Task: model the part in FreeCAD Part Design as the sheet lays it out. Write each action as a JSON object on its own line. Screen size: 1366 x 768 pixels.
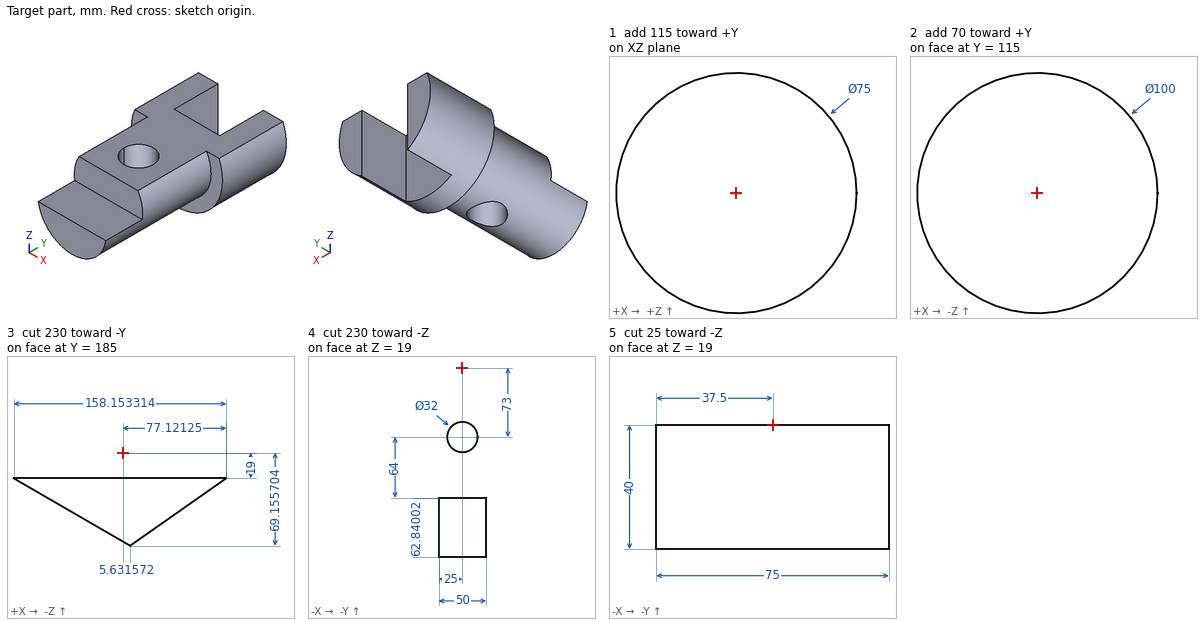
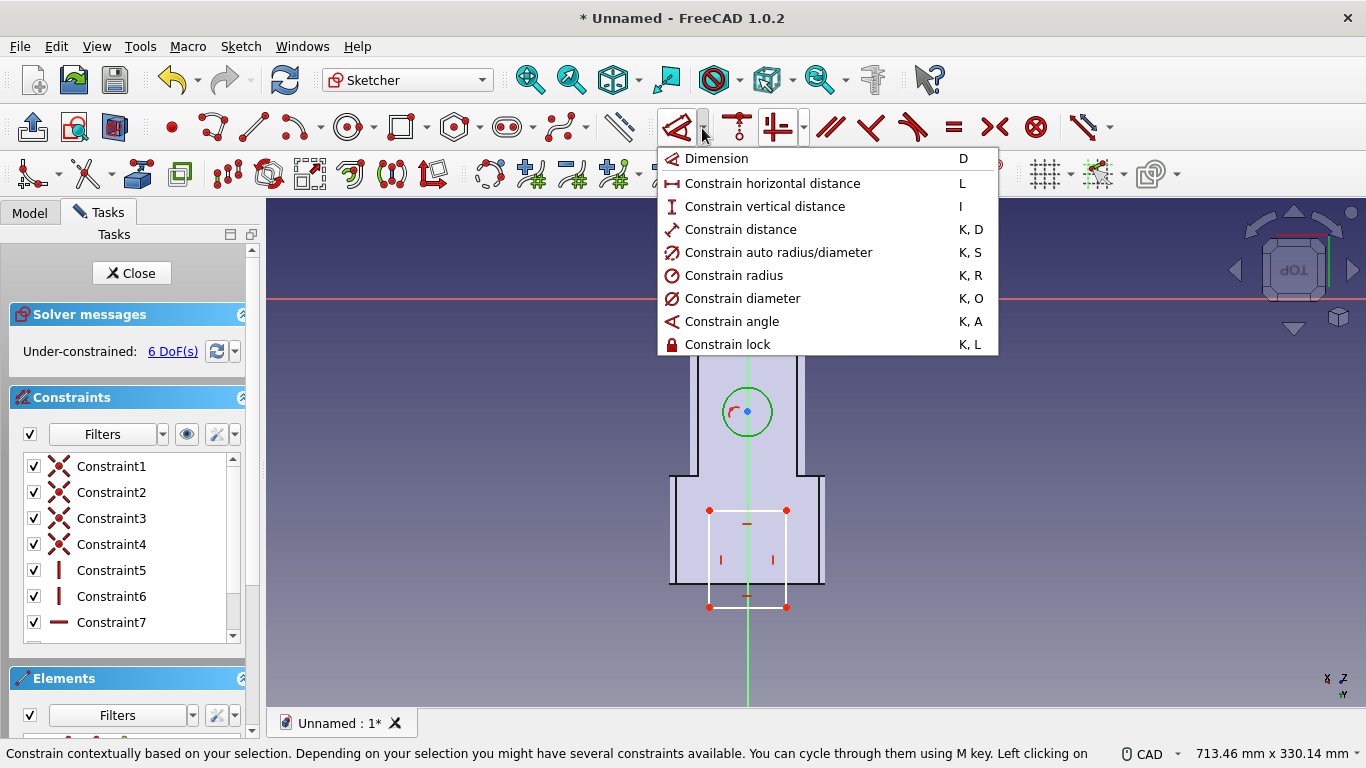
{"action": "left_click", "coordinate": [828, 298]}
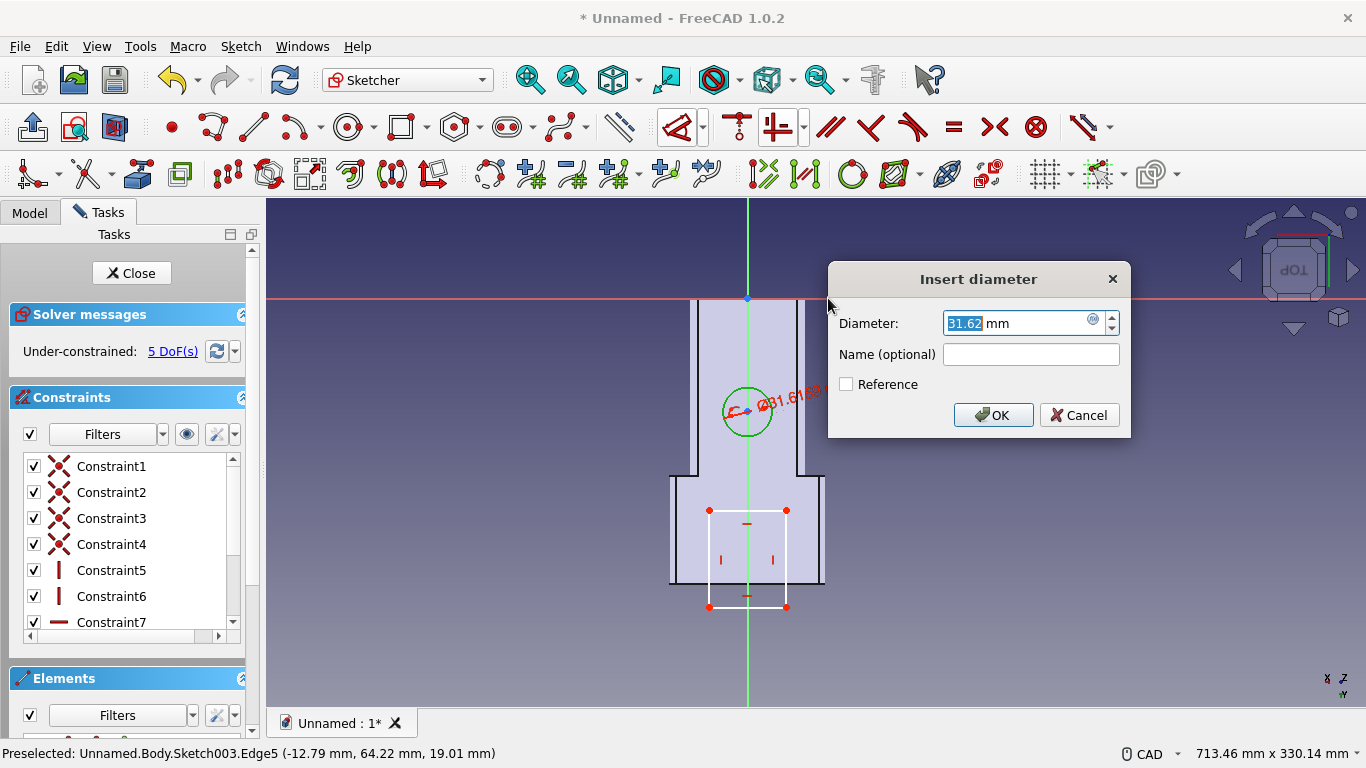
{"action": "type", "text": "32"}
{"action": "key", "text": "Return"}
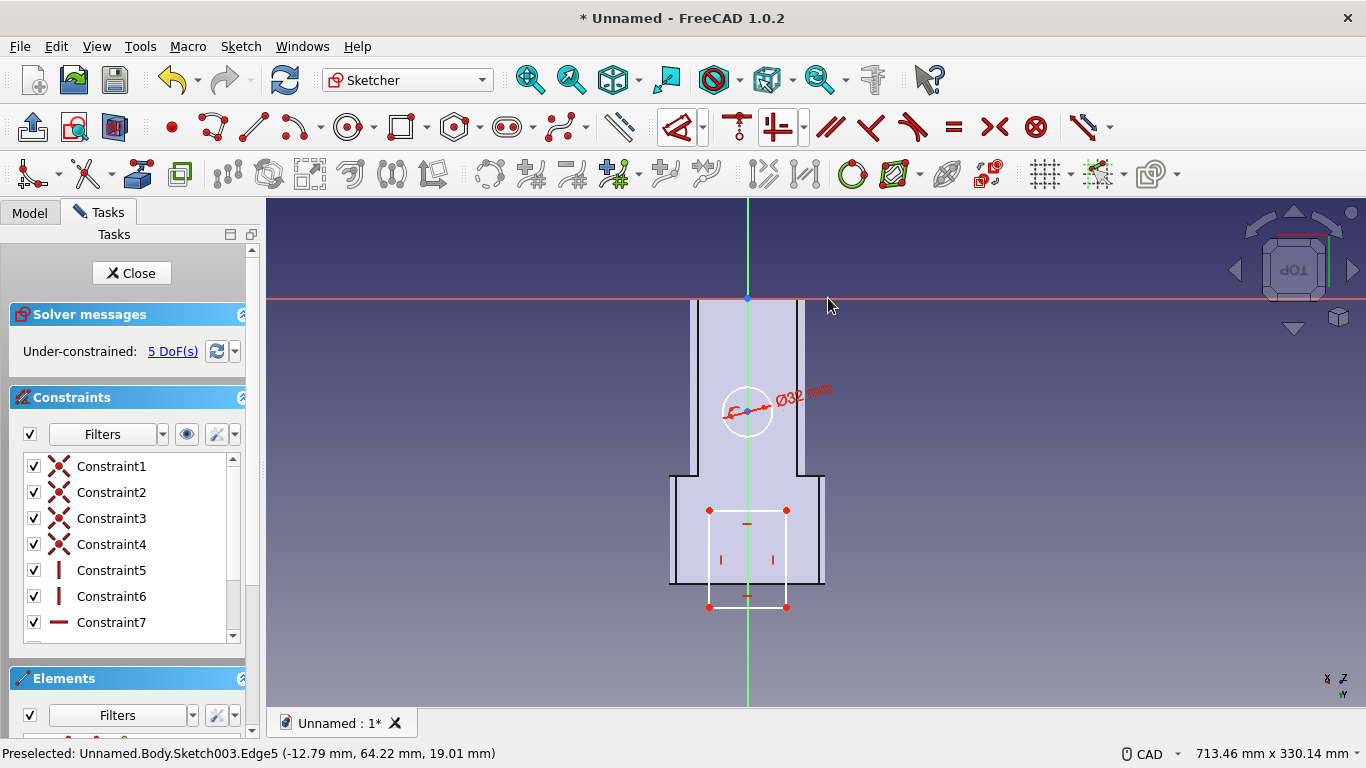
{"action": "left_click", "coordinate": [732, 608]}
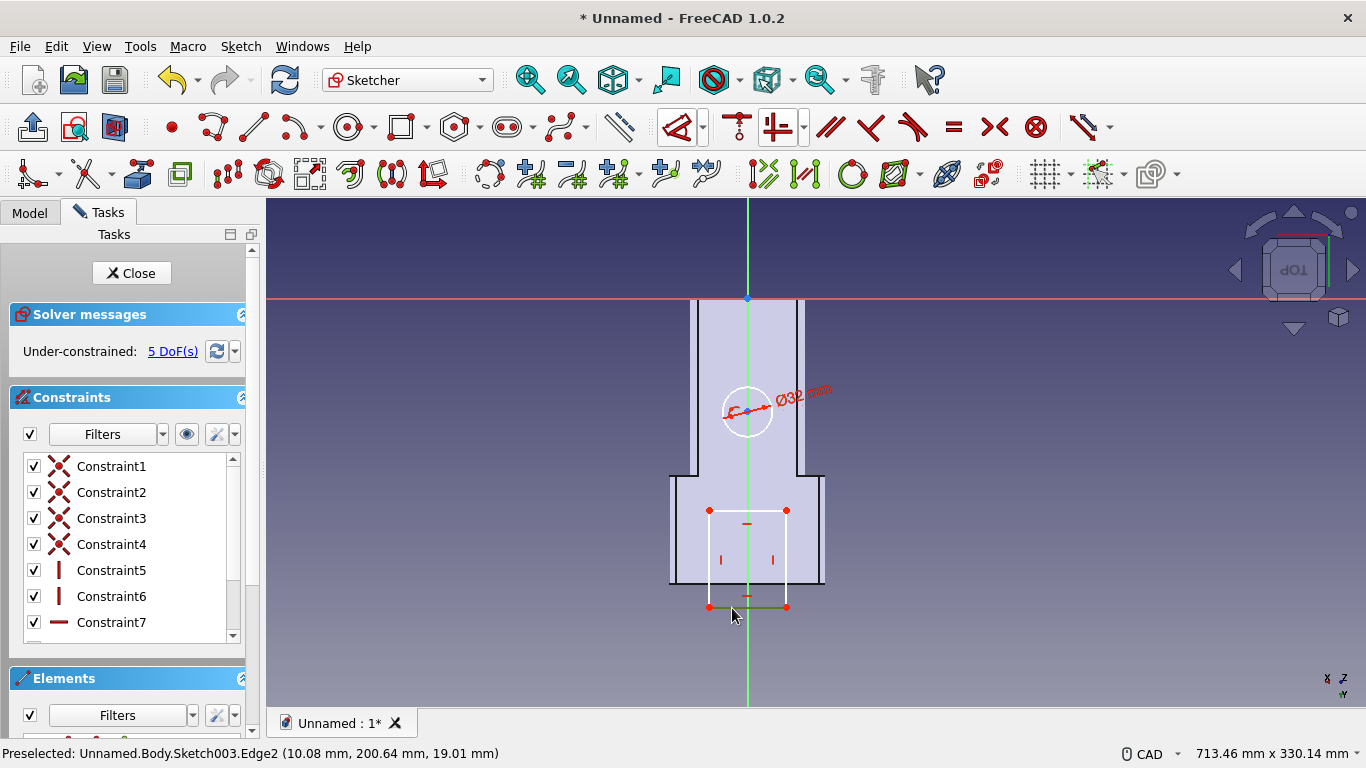
{"action": "key", "text": "l"}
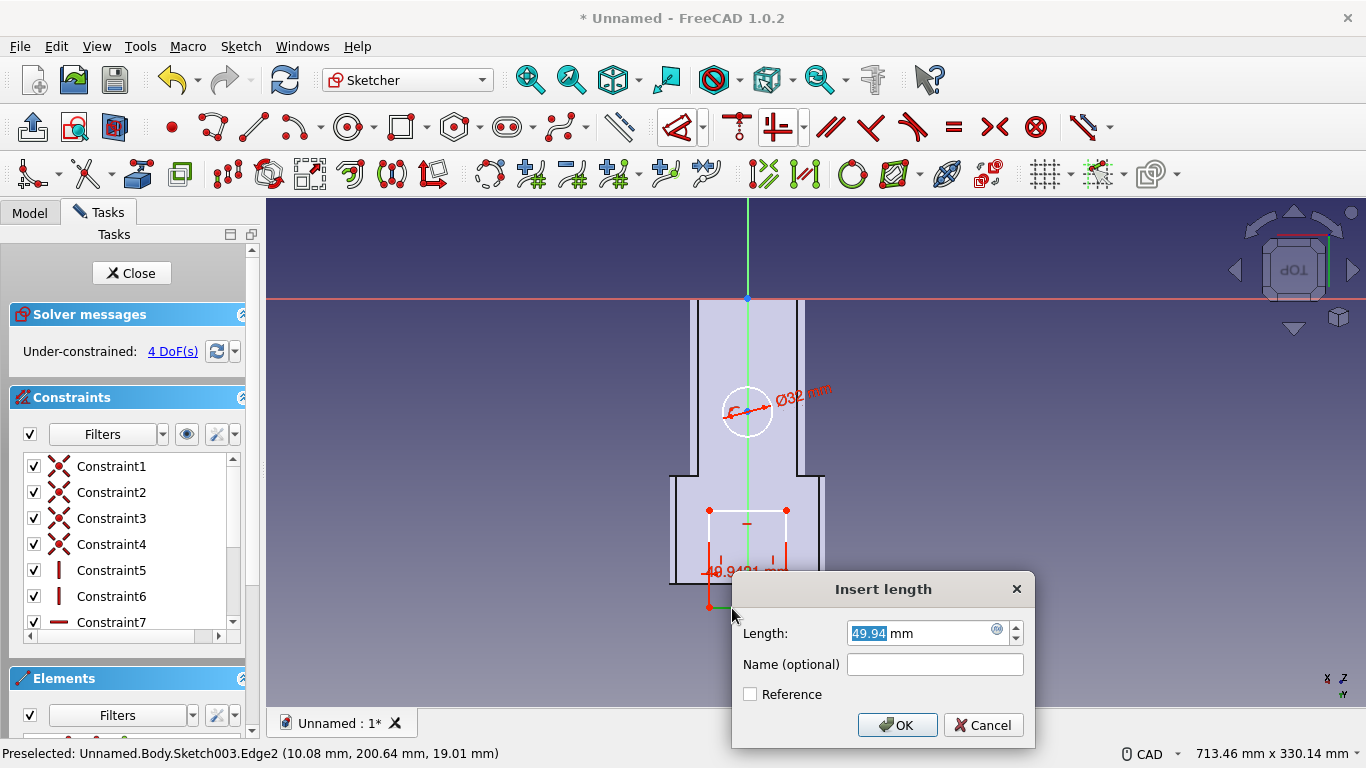
{"action": "type", "text": "50"}
{"action": "key", "text": "Return"}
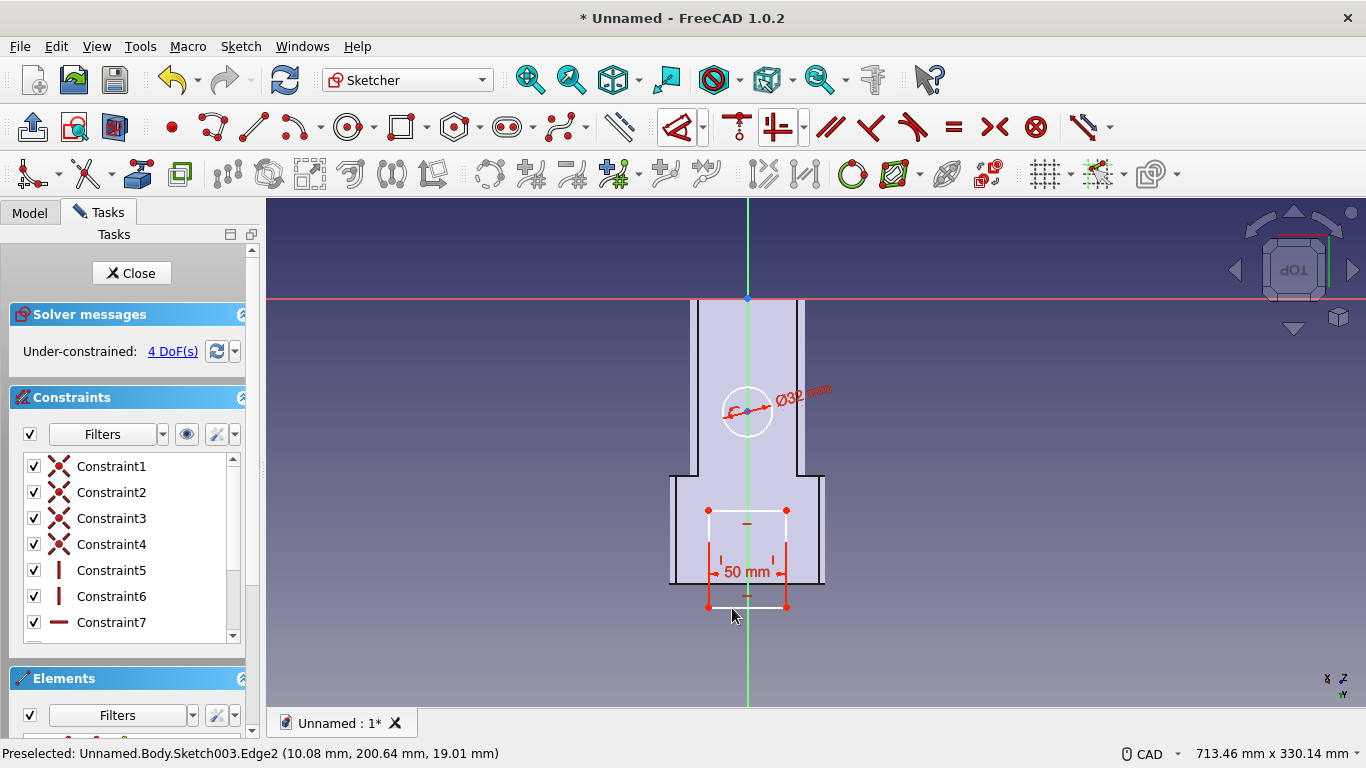
{"action": "left_click", "coordinate": [748, 412]}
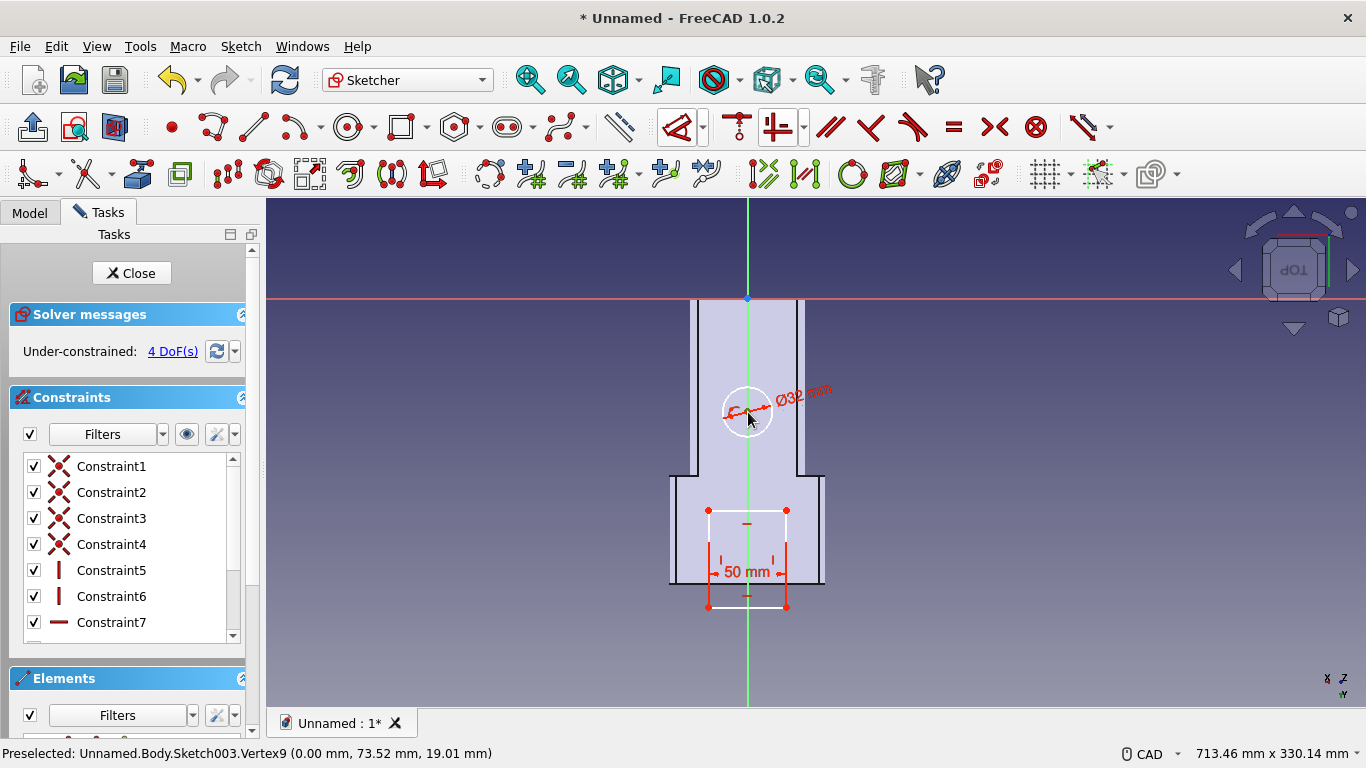
{"action": "left_click", "coordinate": [702, 128]}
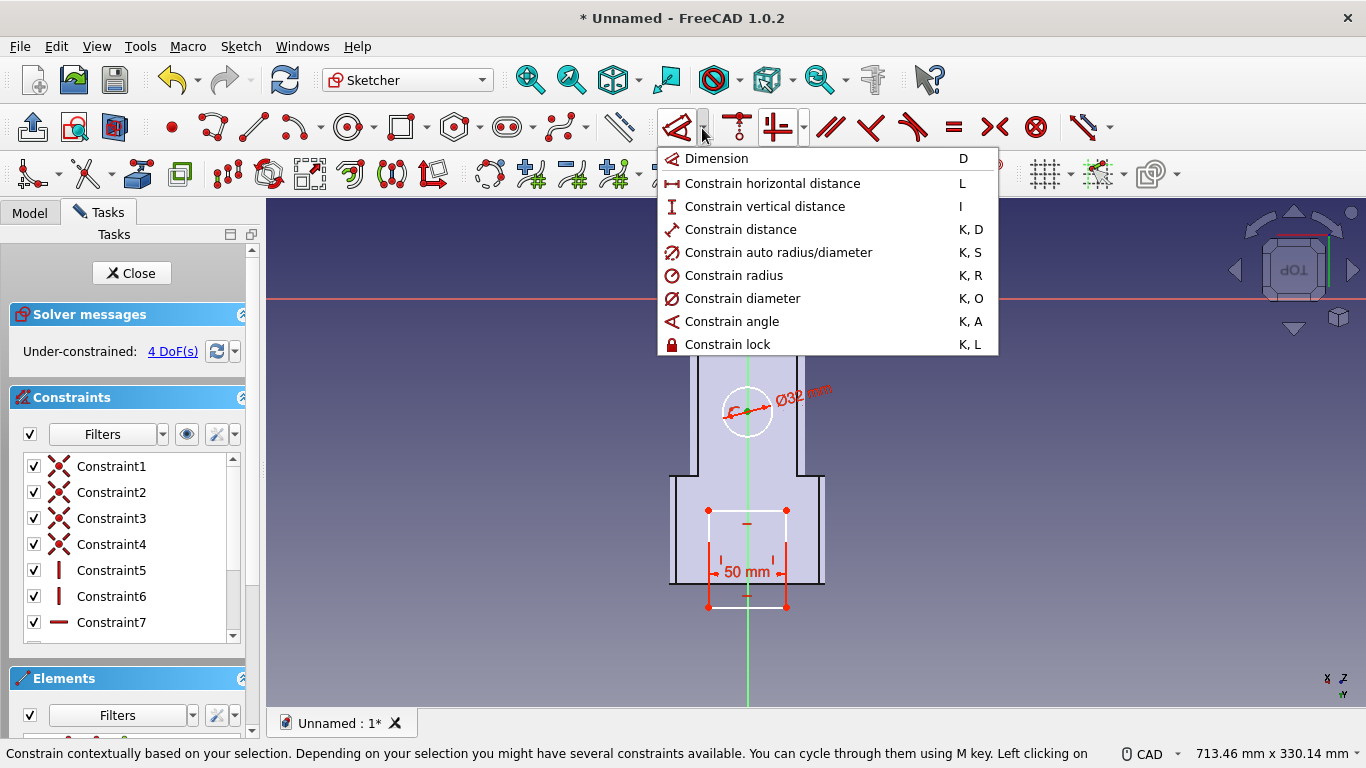
{"action": "left_click", "coordinate": [828, 206]}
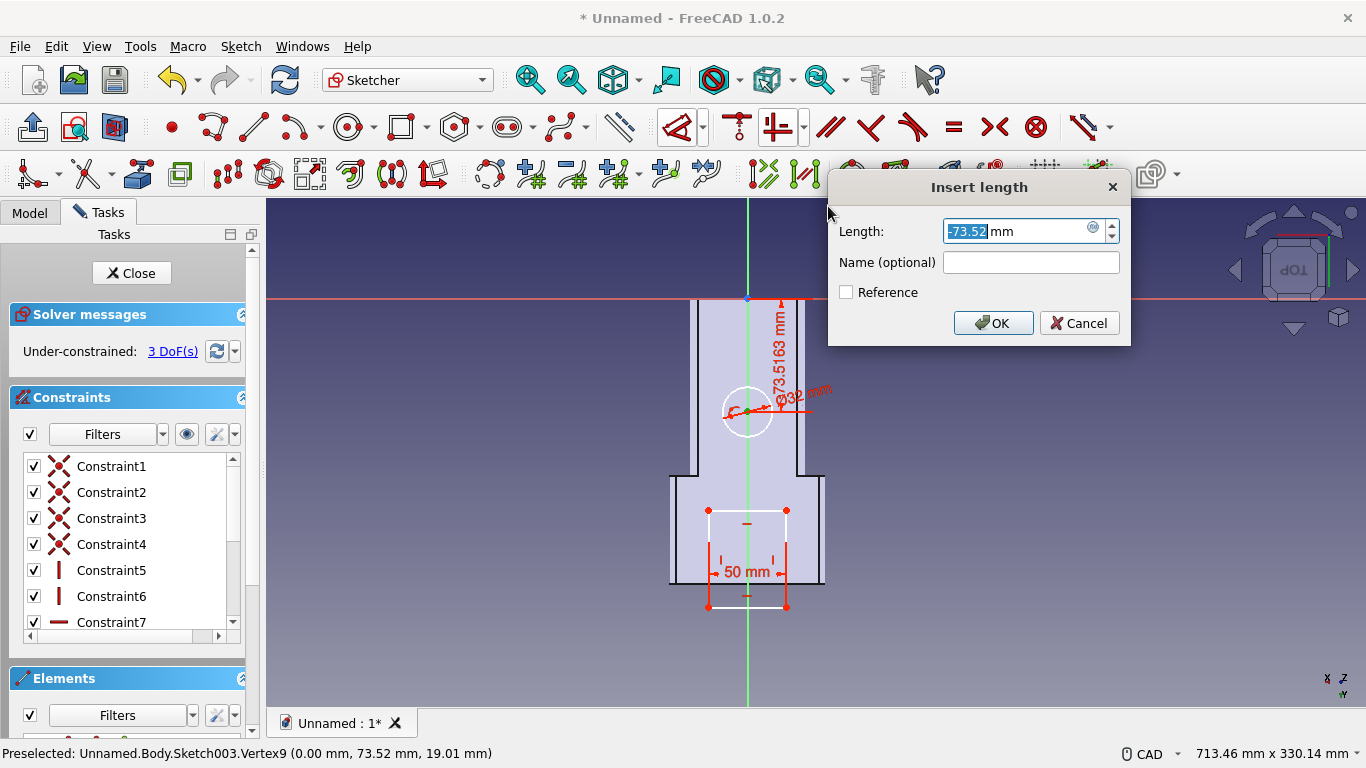
{"action": "type", "text": "-73"}
{"action": "key", "text": "Return"}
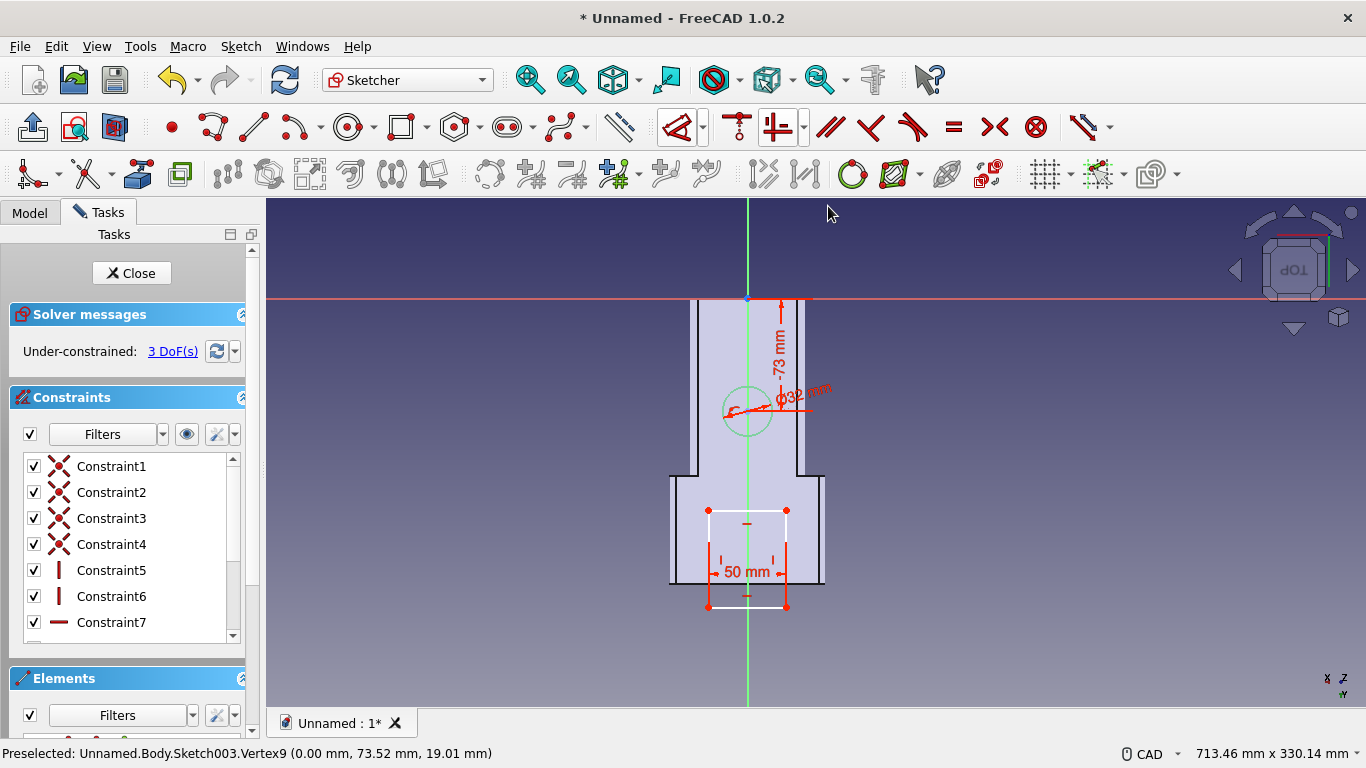
{"action": "left_click", "coordinate": [709, 511]}